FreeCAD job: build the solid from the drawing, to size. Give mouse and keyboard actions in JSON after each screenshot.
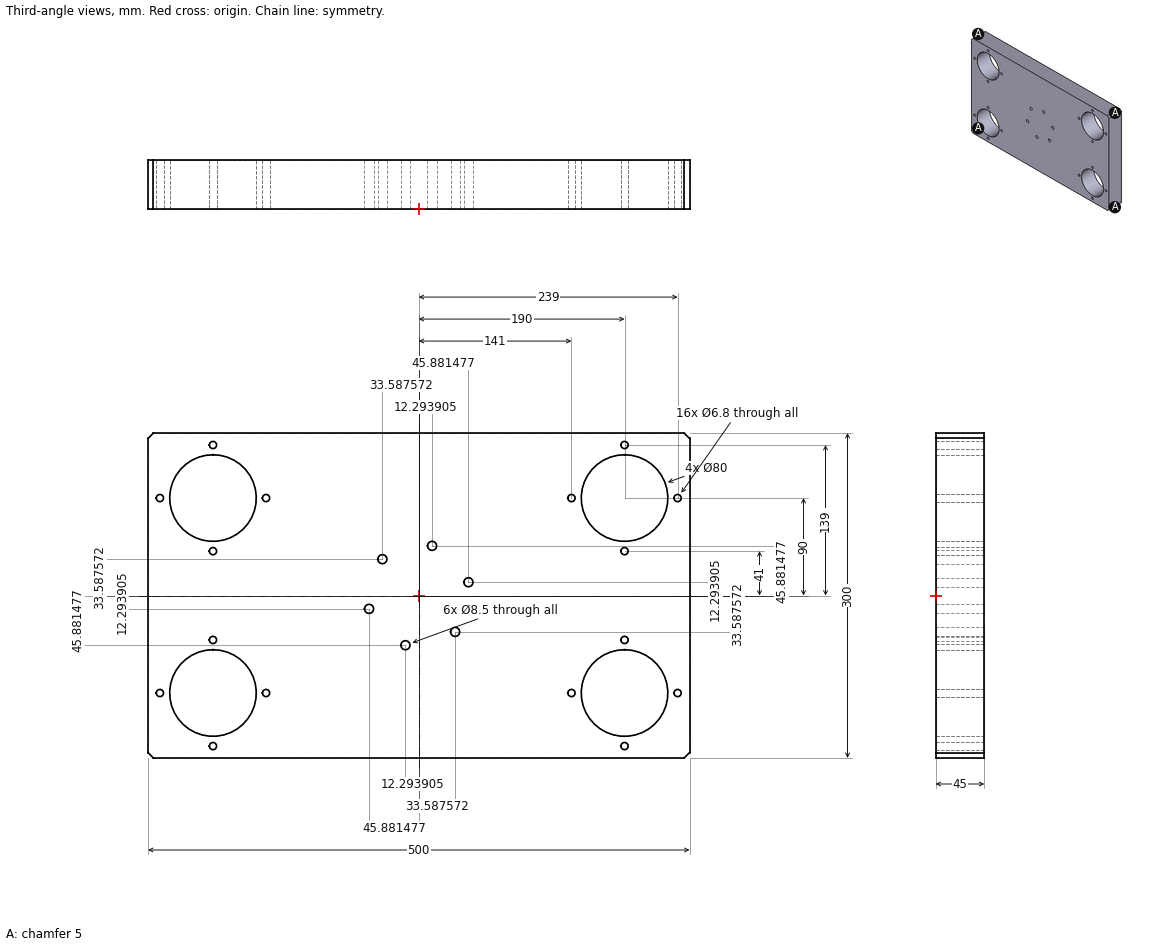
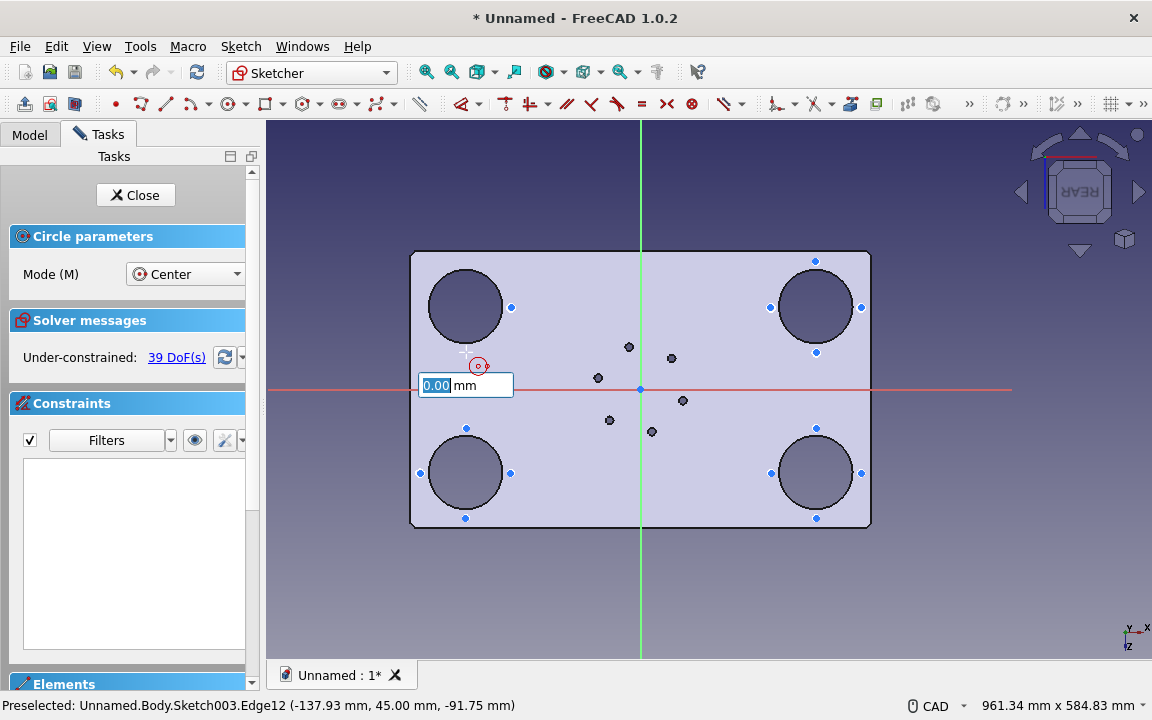
{"action": "scroll", "coordinate": [468, 349], "scroll_direction": "up", "scroll_amount": 9}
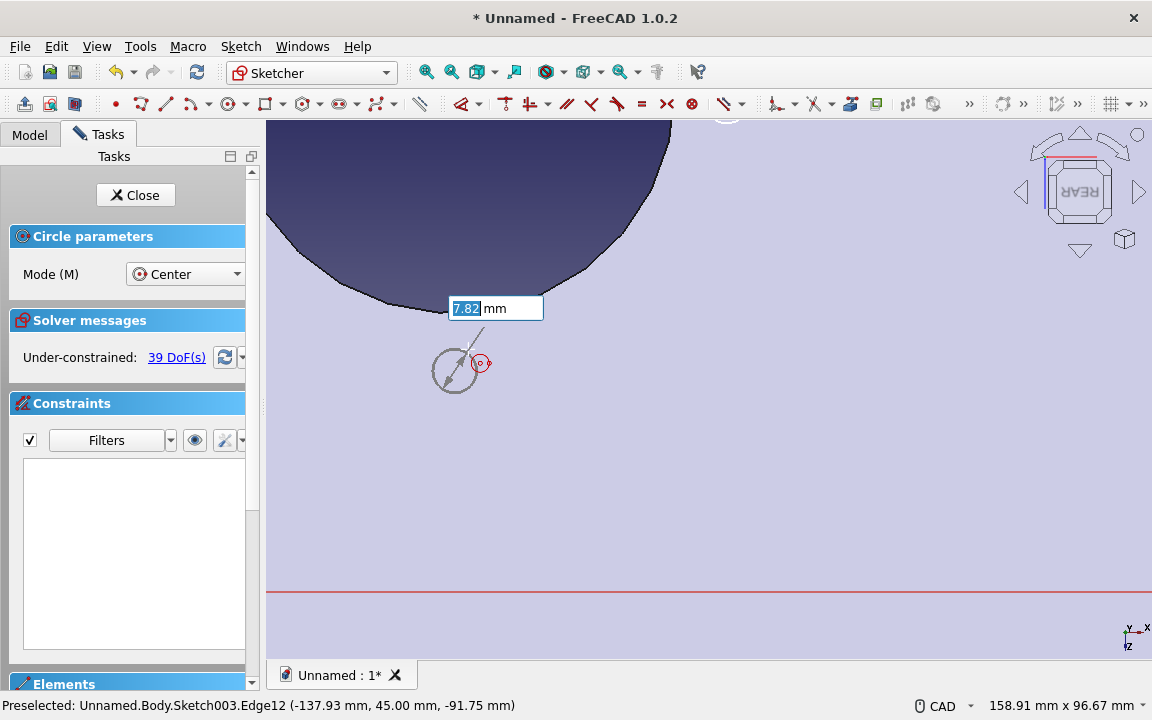
{"action": "left_click", "coordinate": [465, 350]}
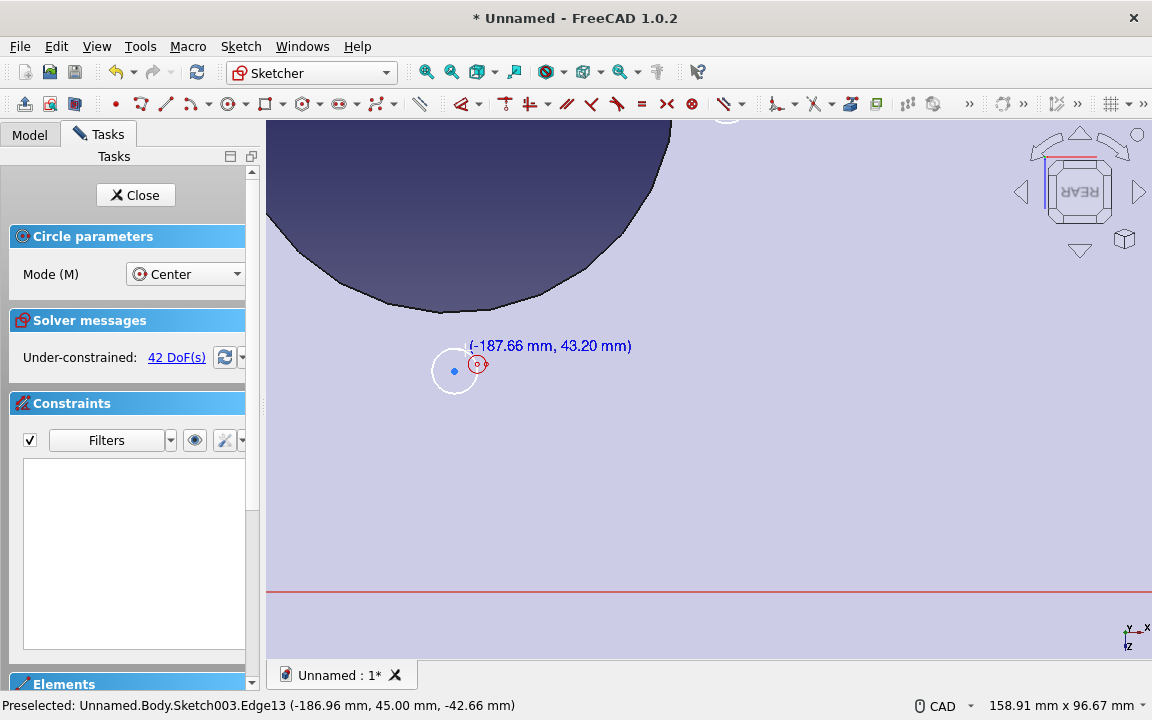
{"action": "scroll", "coordinate": [468, 349], "scroll_direction": "down", "scroll_amount": 9}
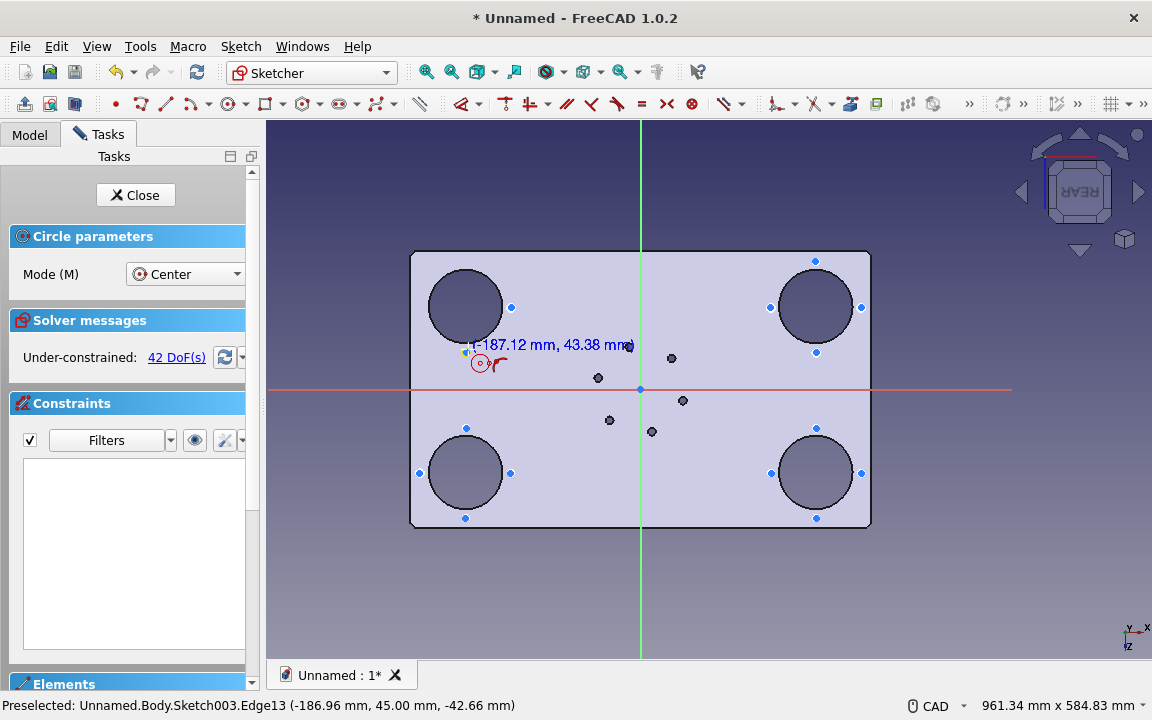
{"action": "scroll", "coordinate": [420, 307], "scroll_direction": "up", "scroll_amount": 10}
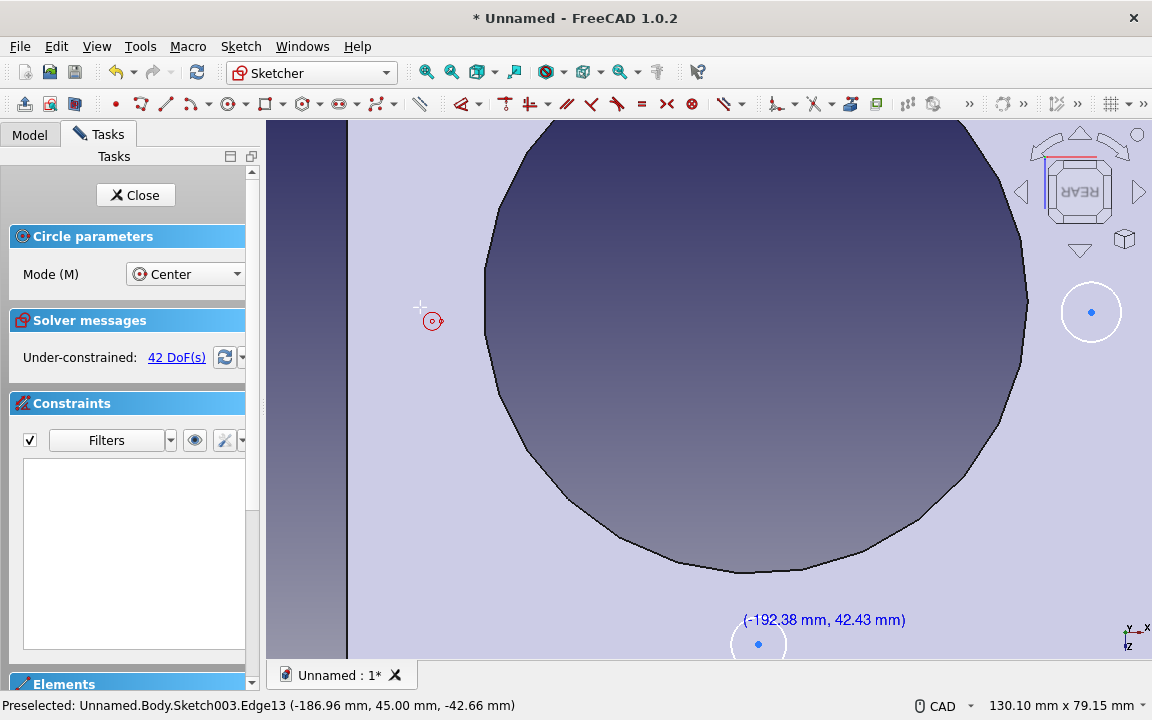
{"action": "scroll", "coordinate": [420, 307], "scroll_direction": "down", "scroll_amount": 10}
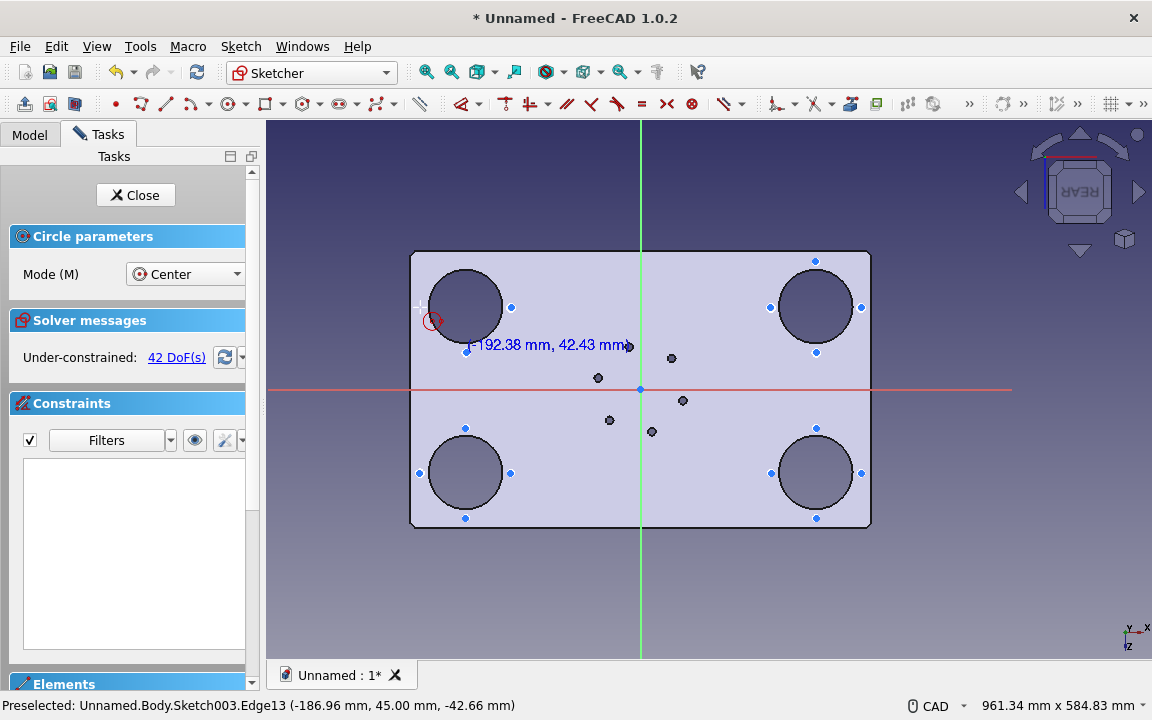
{"action": "left_click", "coordinate": [420, 307]}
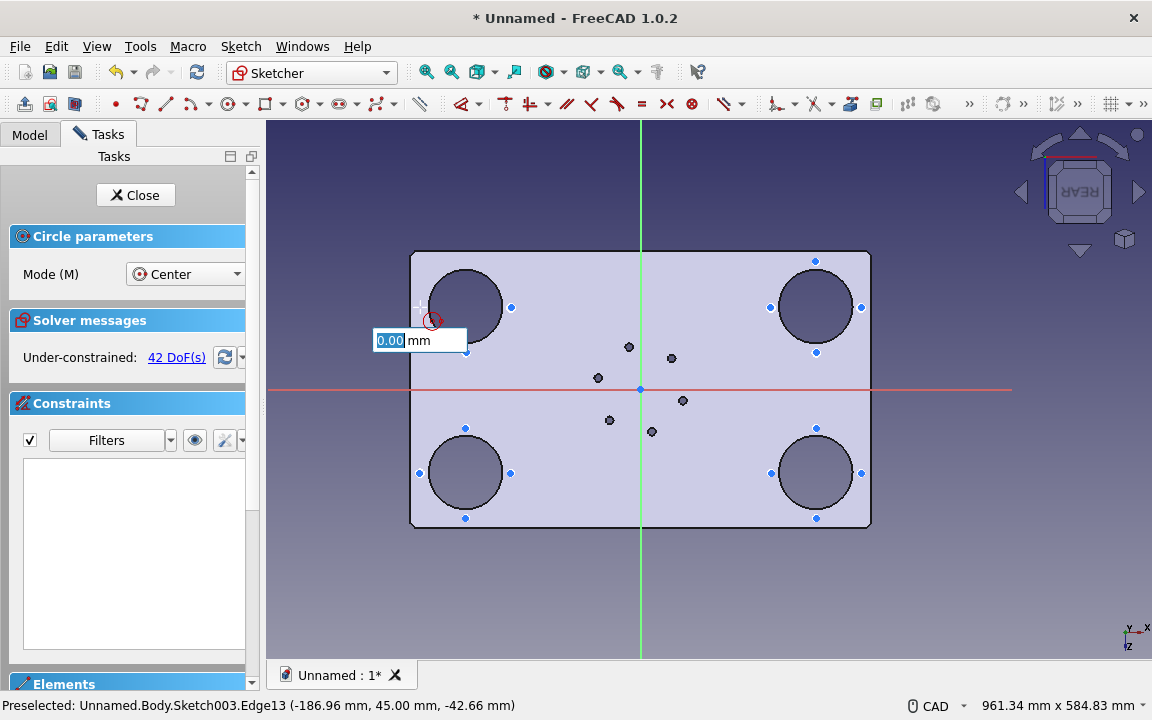
{"action": "scroll", "coordinate": [423, 304], "scroll_direction": "up", "scroll_amount": 9}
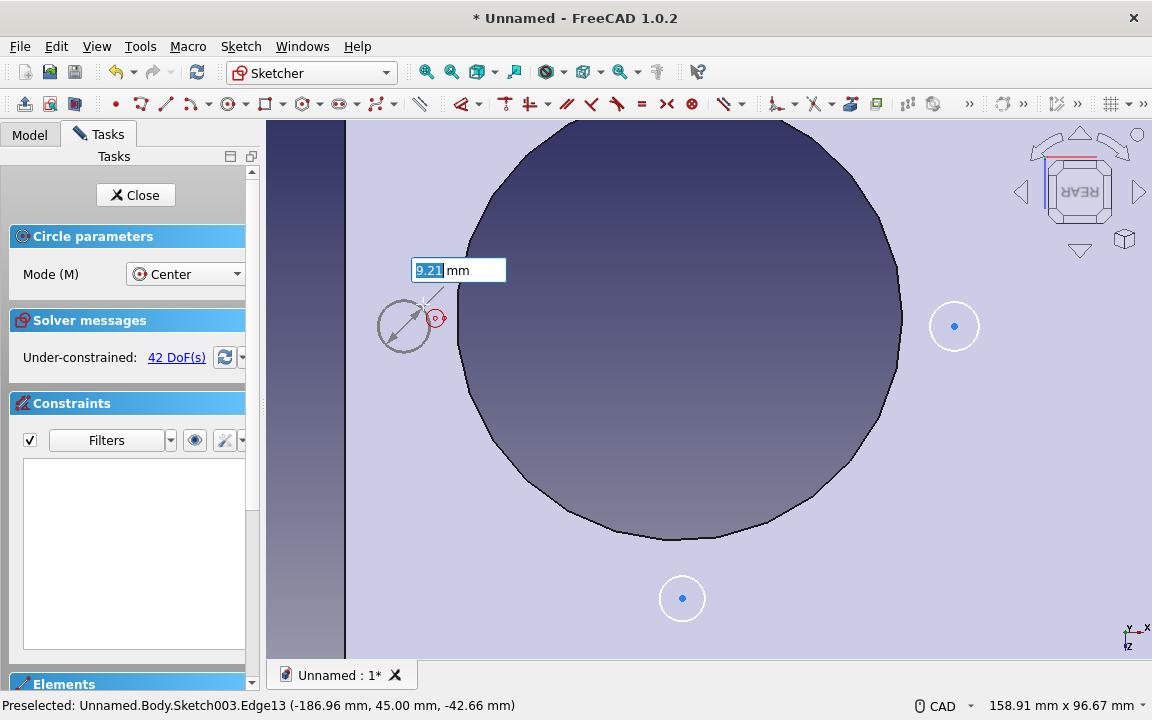
{"action": "left_click", "coordinate": [420, 304]}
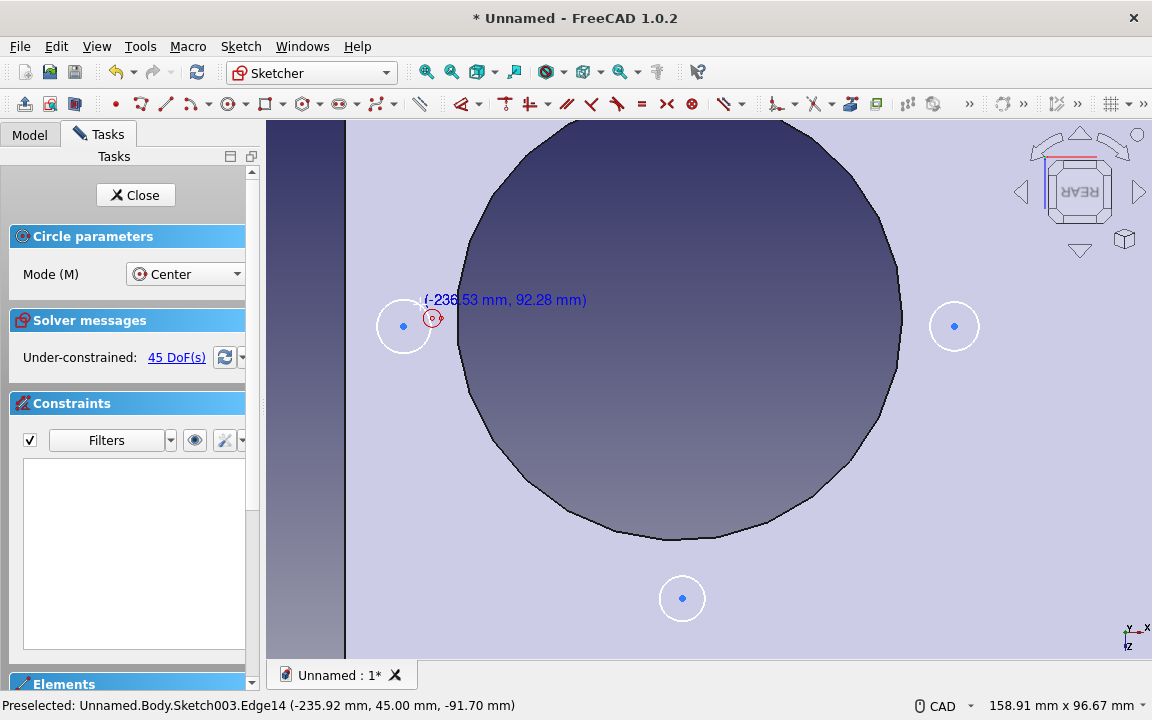
{"action": "scroll", "coordinate": [423, 304], "scroll_direction": "down", "scroll_amount": 9}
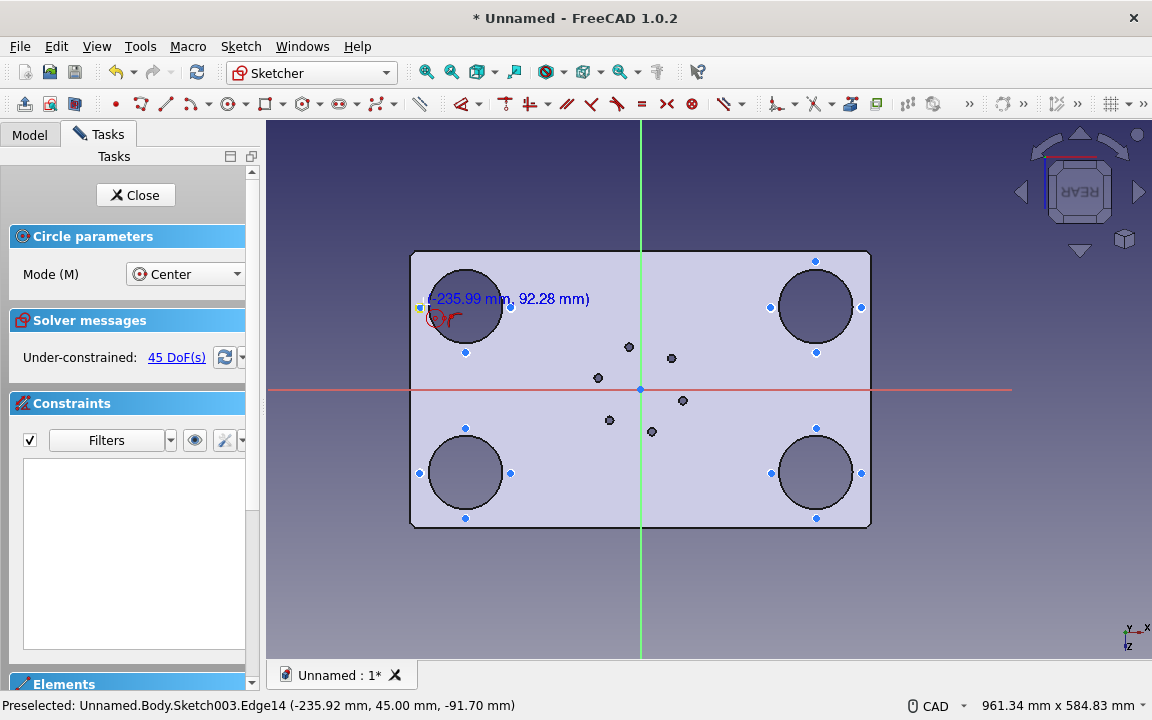
{"action": "scroll", "coordinate": [466, 261], "scroll_direction": "up", "scroll_amount": 10}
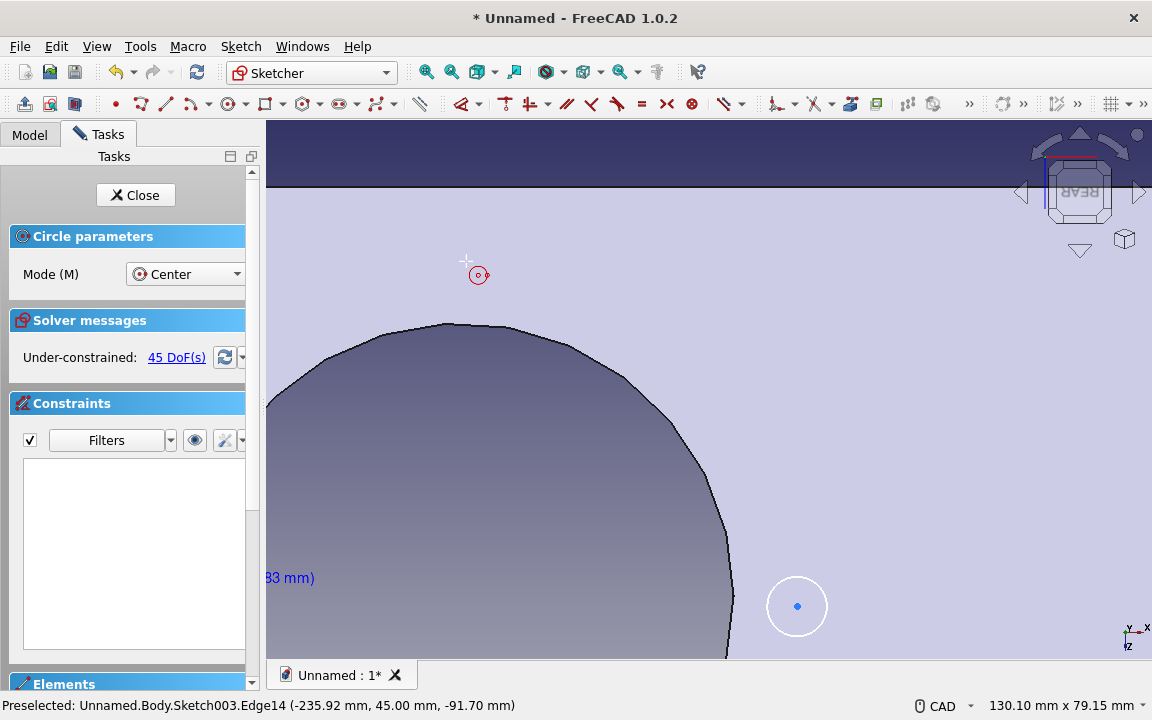
{"action": "scroll", "coordinate": [466, 261], "scroll_direction": "down", "scroll_amount": 10}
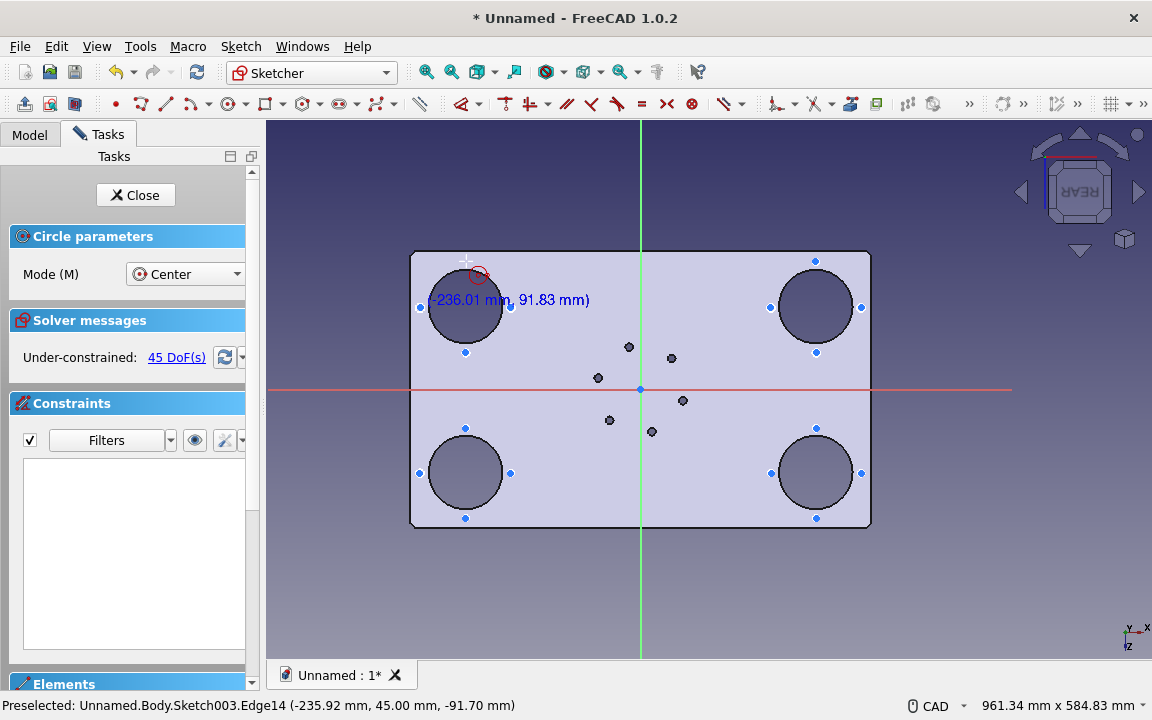
{"action": "left_click", "coordinate": [466, 261]}